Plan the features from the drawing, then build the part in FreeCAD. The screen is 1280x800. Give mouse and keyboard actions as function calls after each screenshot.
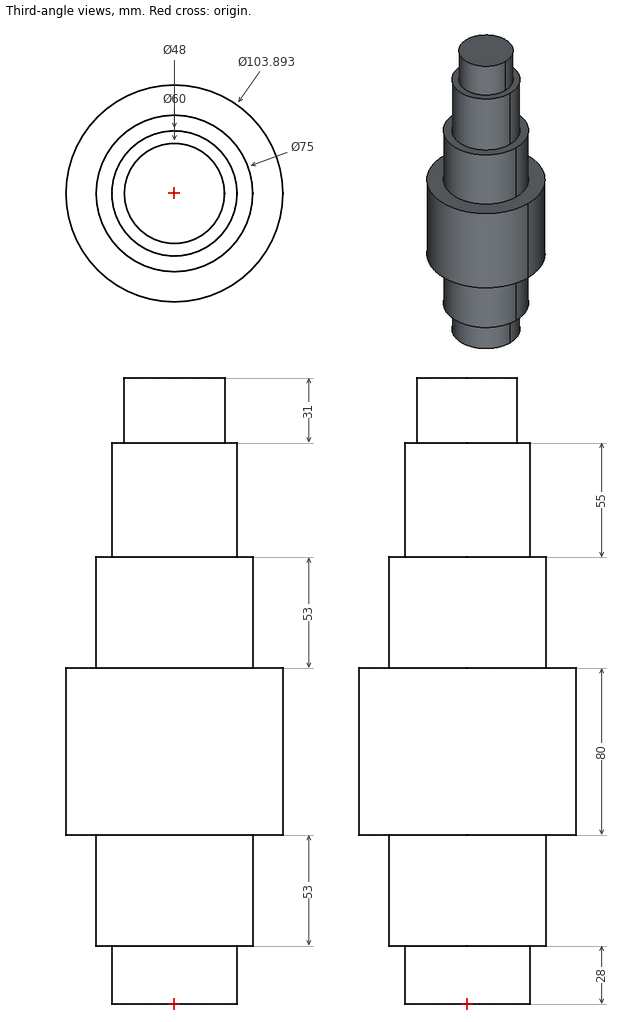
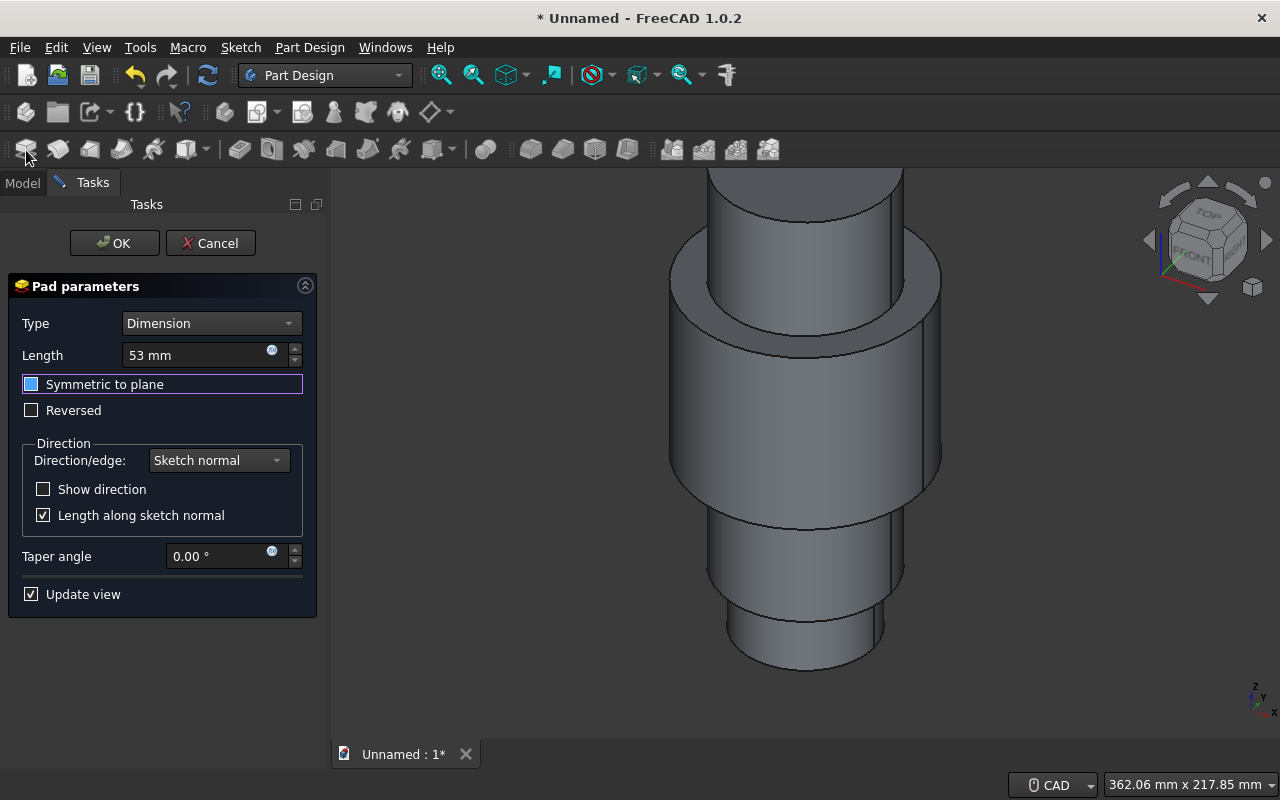
click(115, 243)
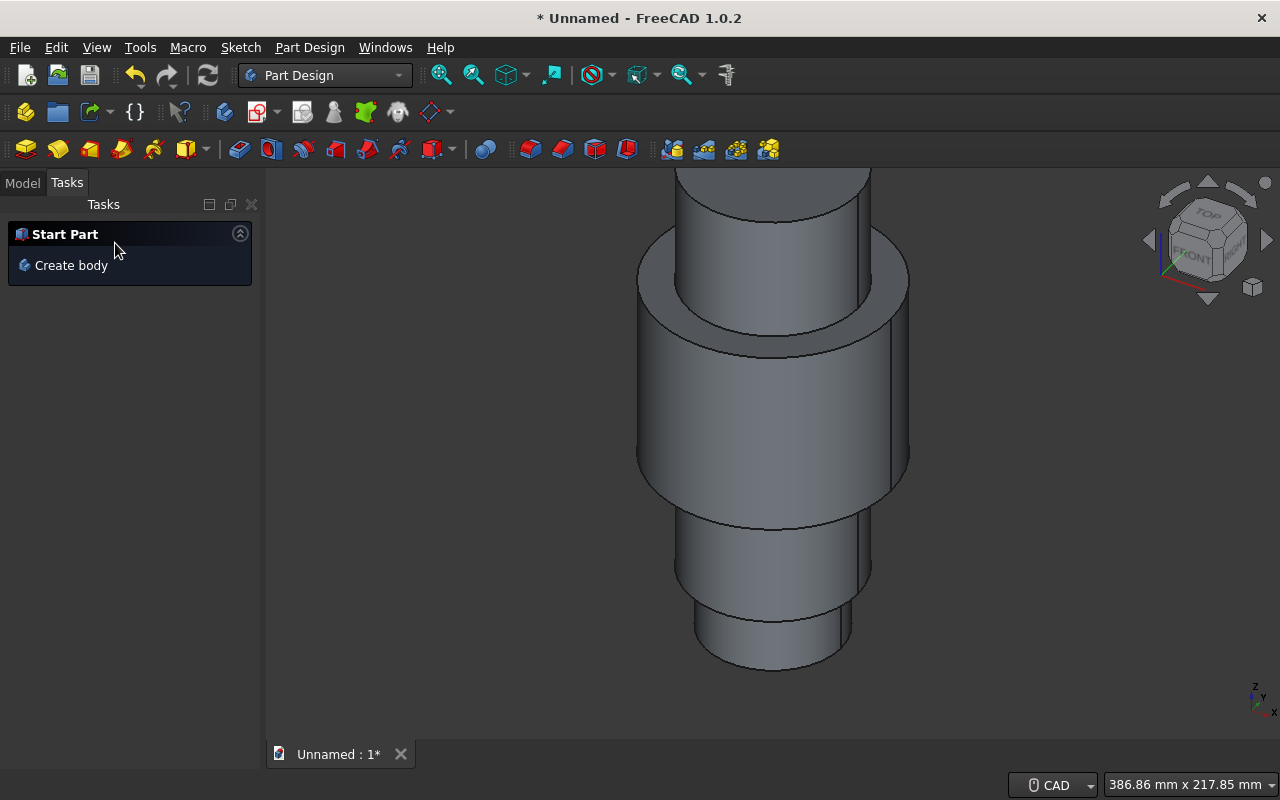
click(442, 76)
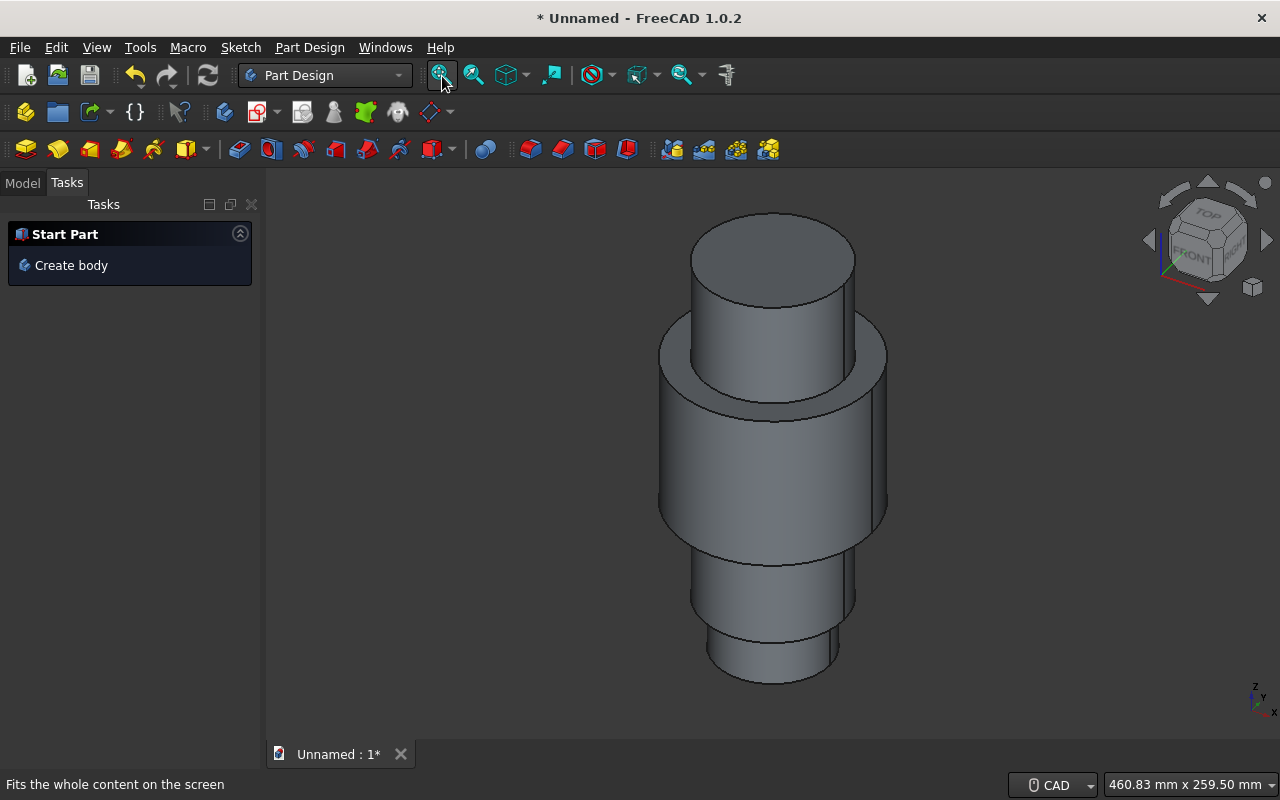
click(773, 260)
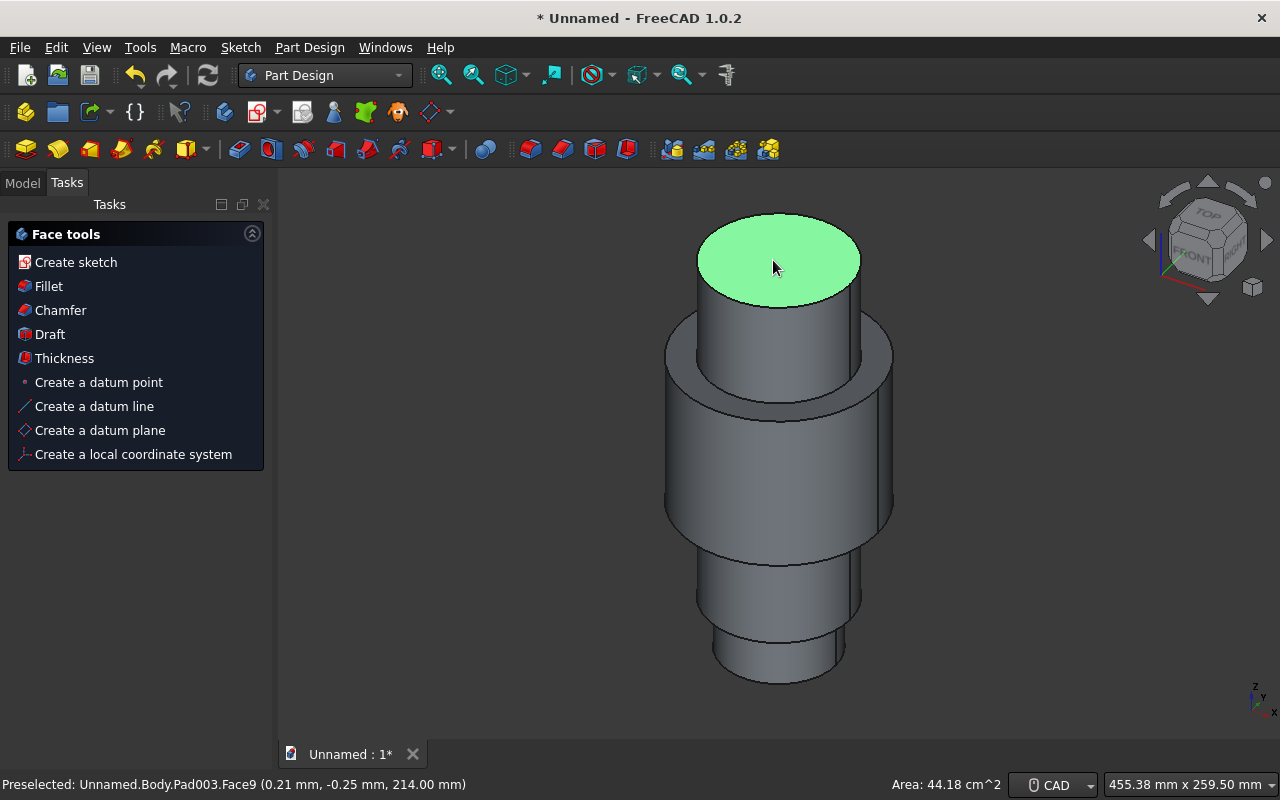
click(258, 112)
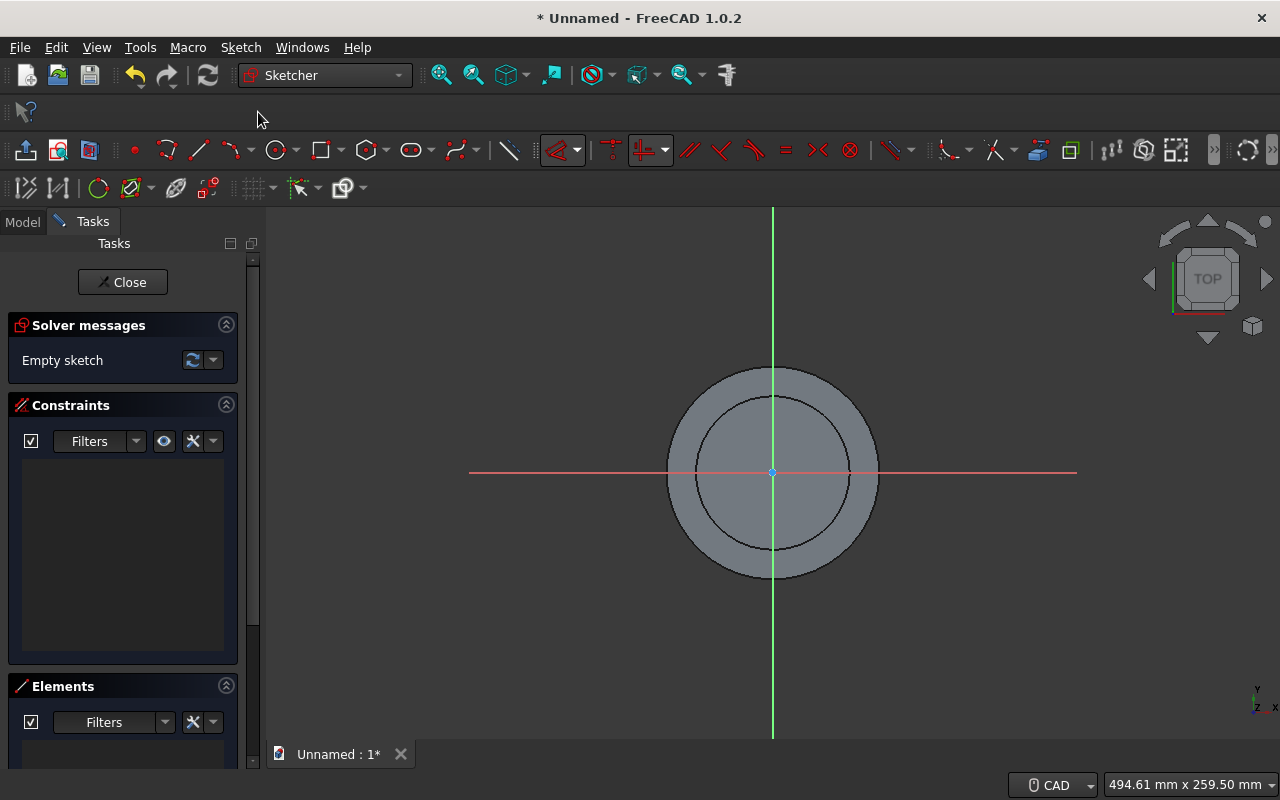
scroll(813, 473, up, 5)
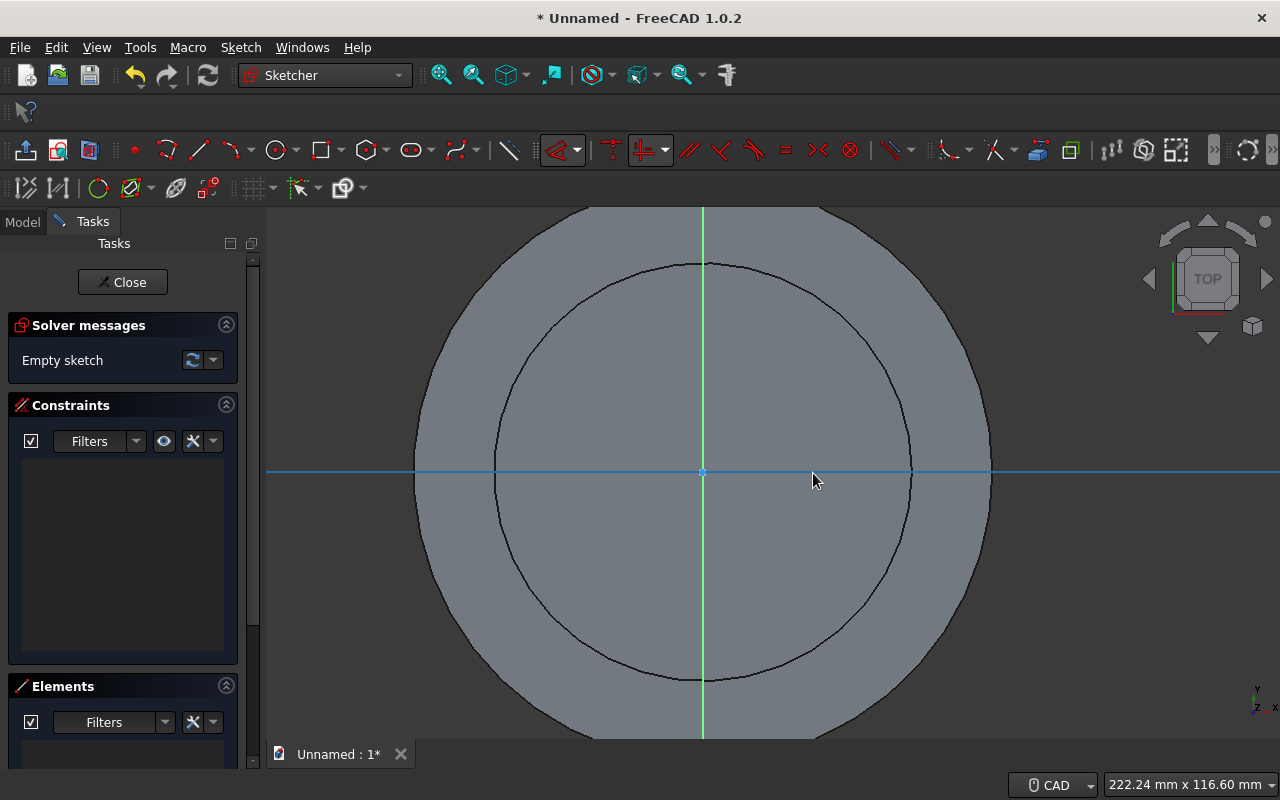
click(276, 150)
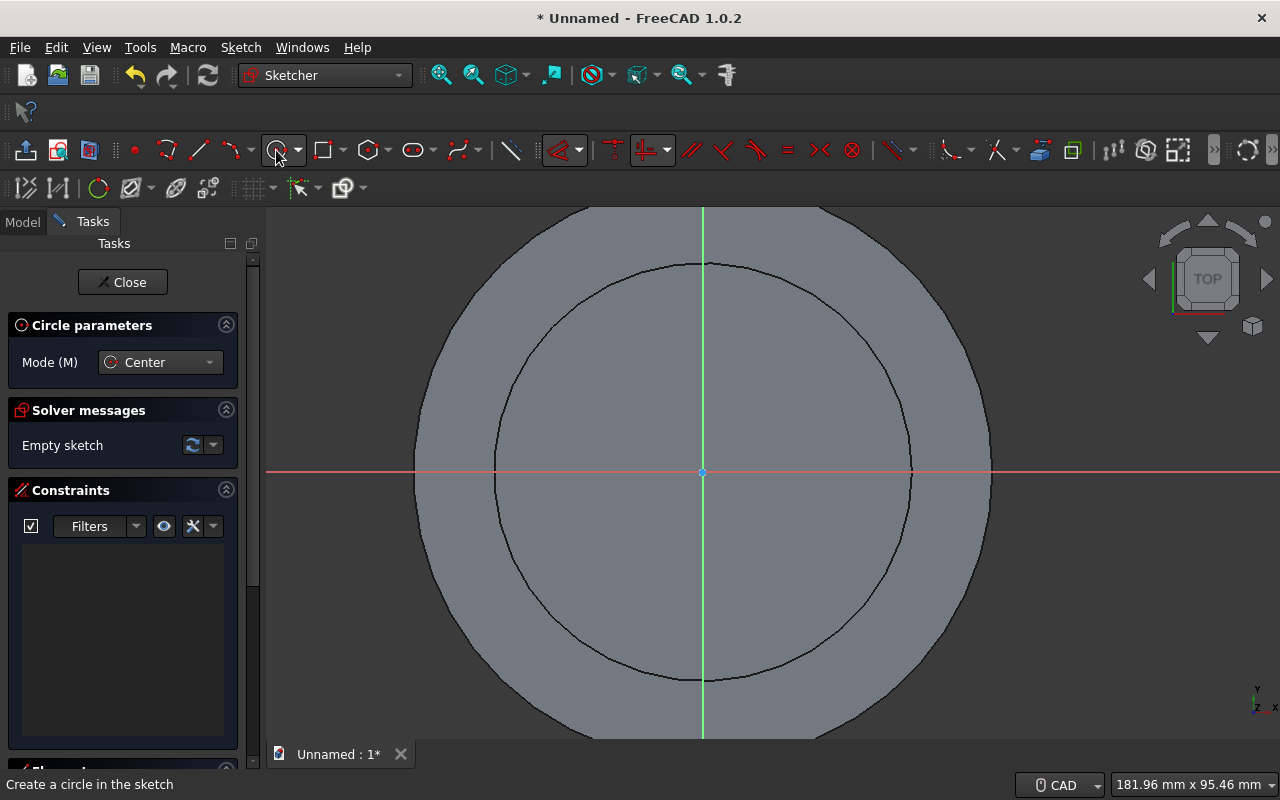
click(703, 472)
move(821, 354)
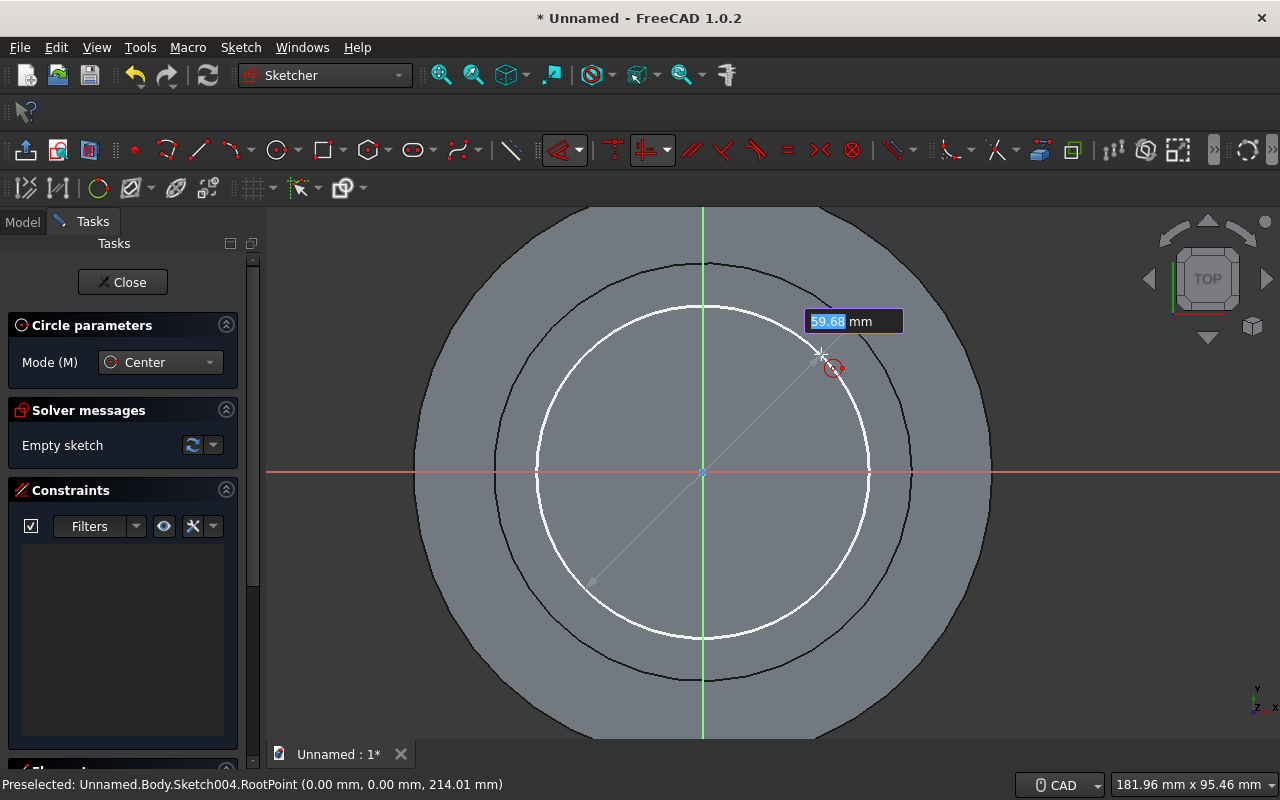
text(60)
key(Return)
key(Escape)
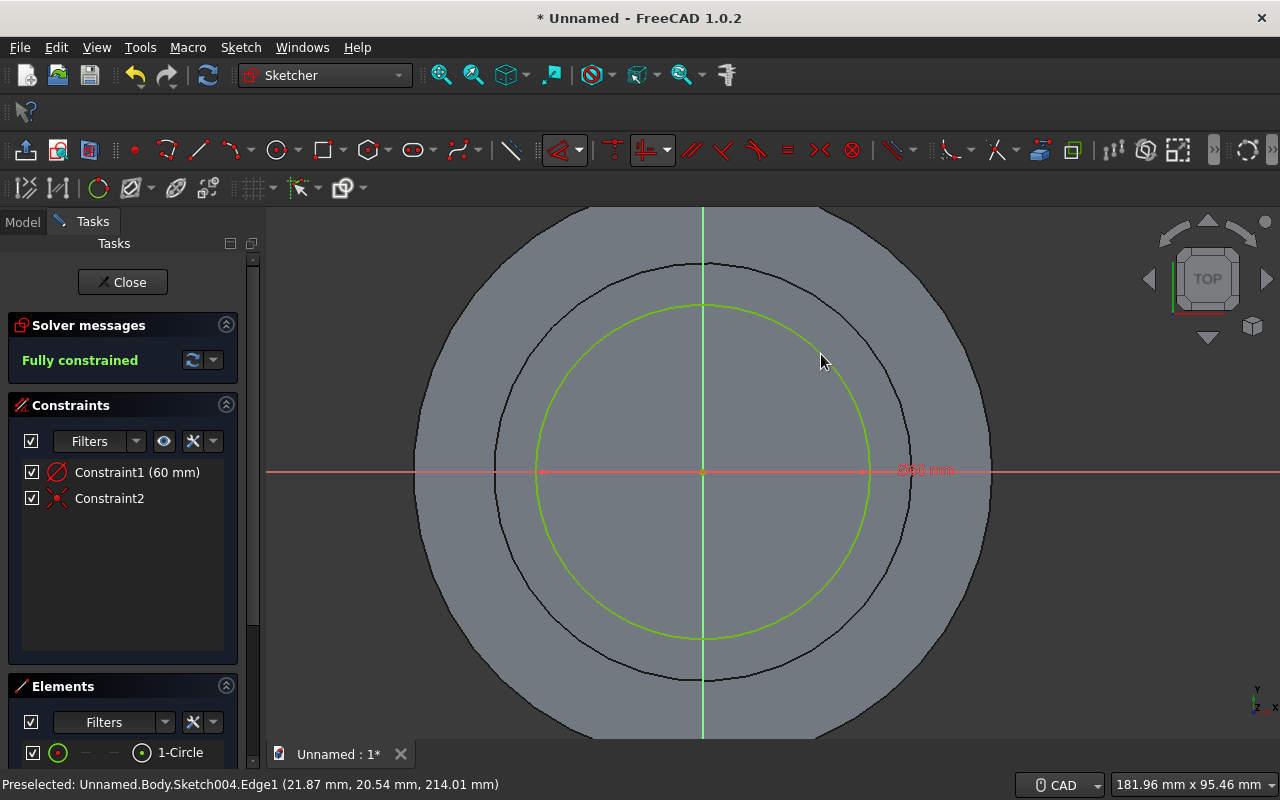
click(123, 282)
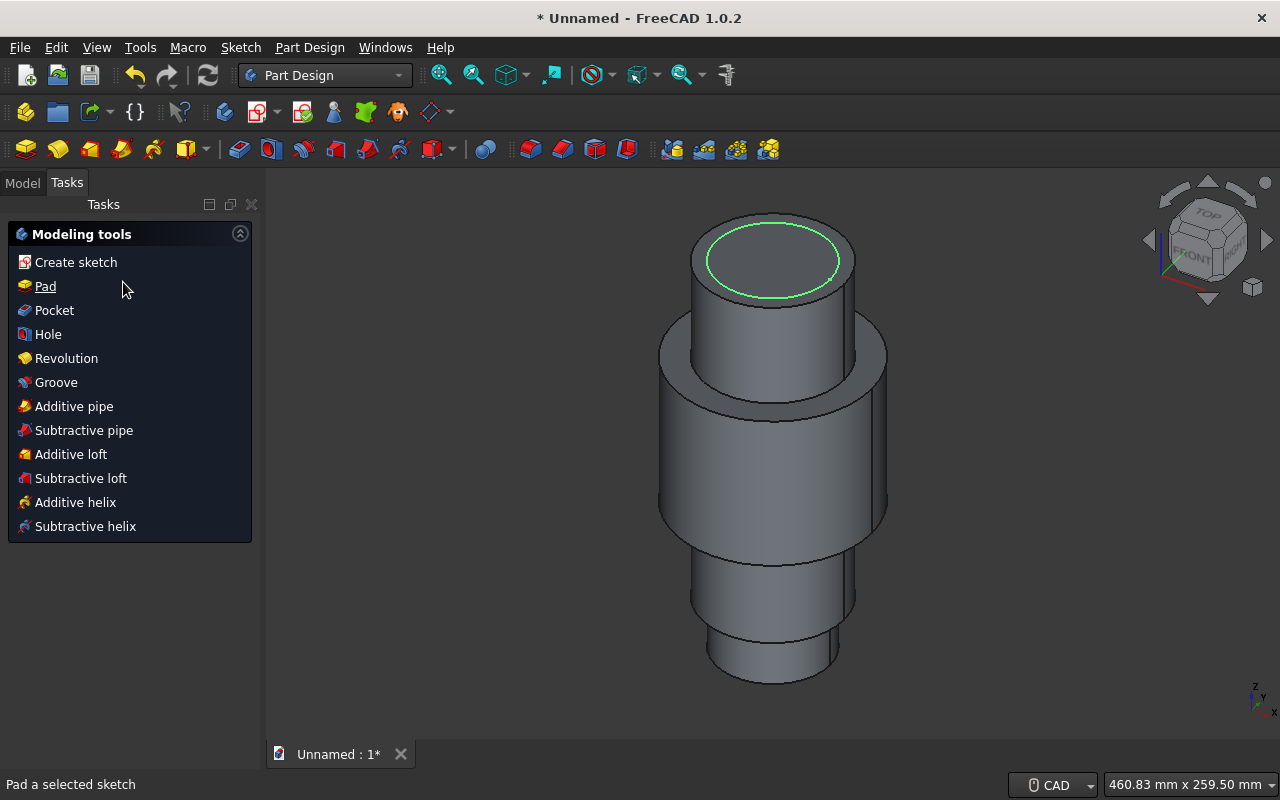
click(26, 150)